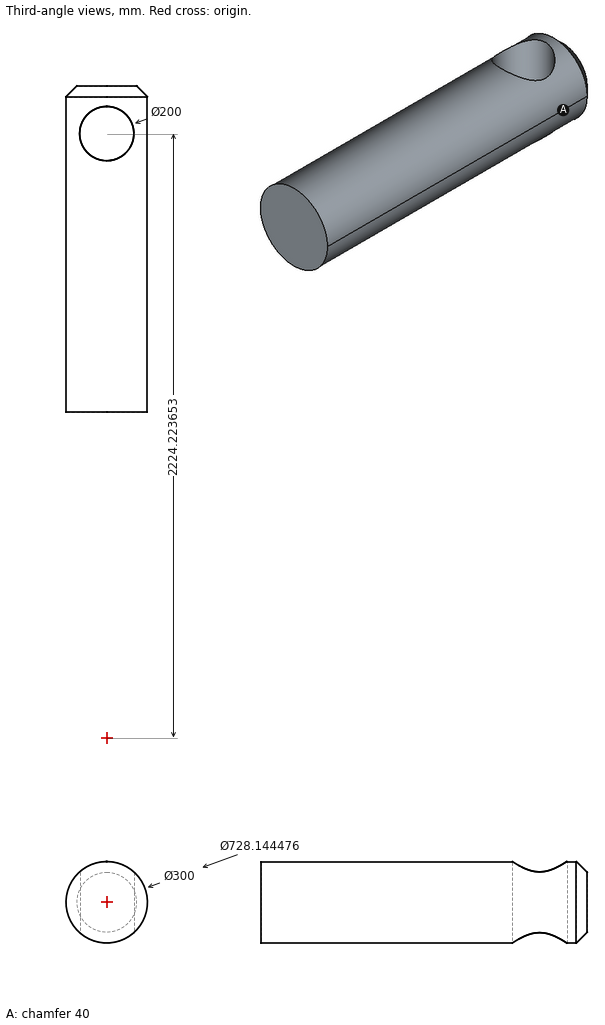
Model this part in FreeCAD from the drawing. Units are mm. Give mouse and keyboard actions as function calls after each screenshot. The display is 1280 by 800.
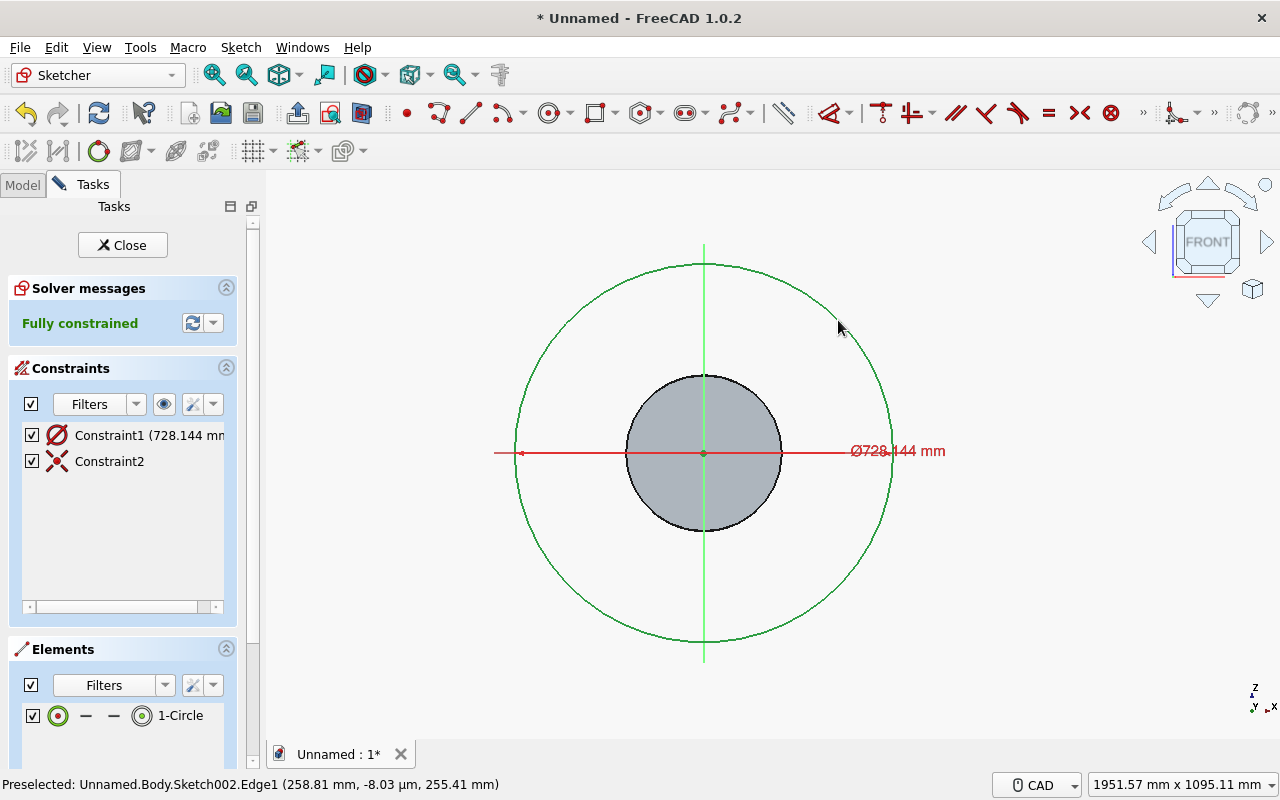
click(123, 245)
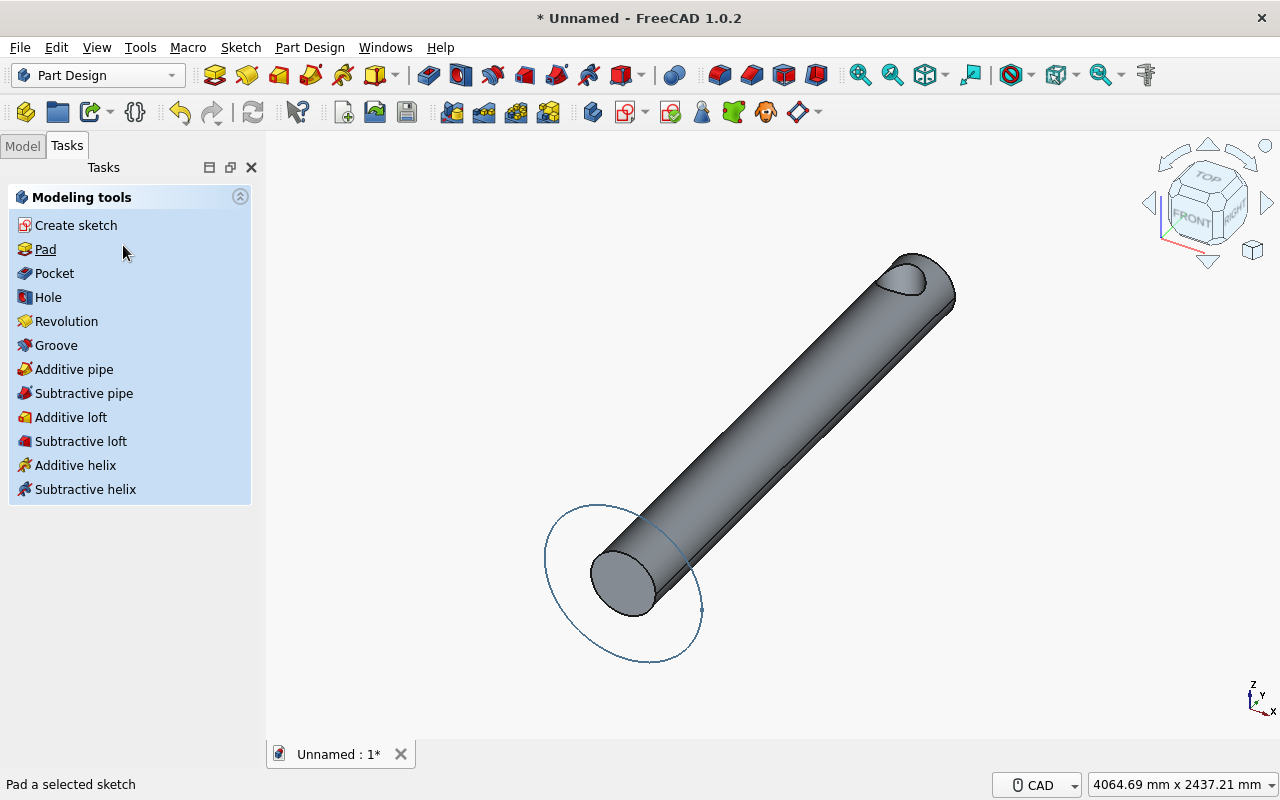
click(430, 76)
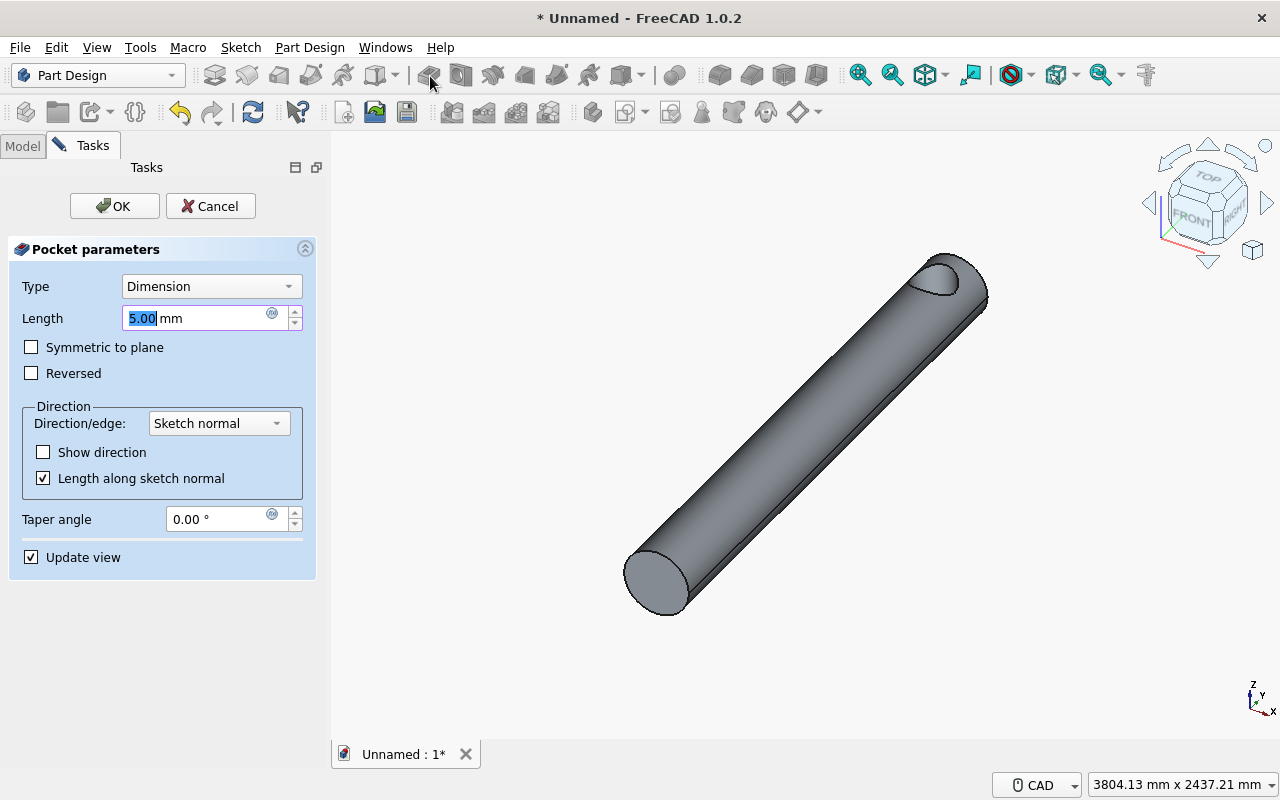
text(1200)
key(Tab)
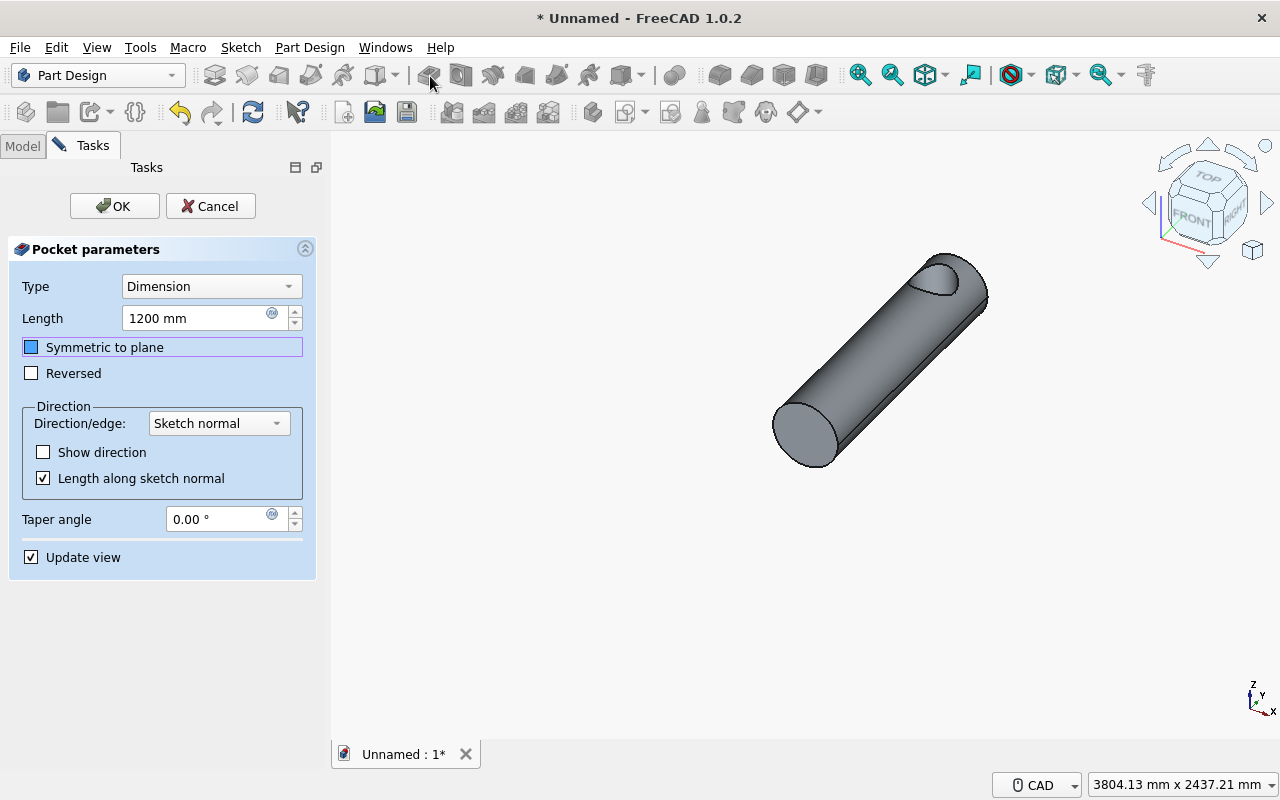
click(115, 206)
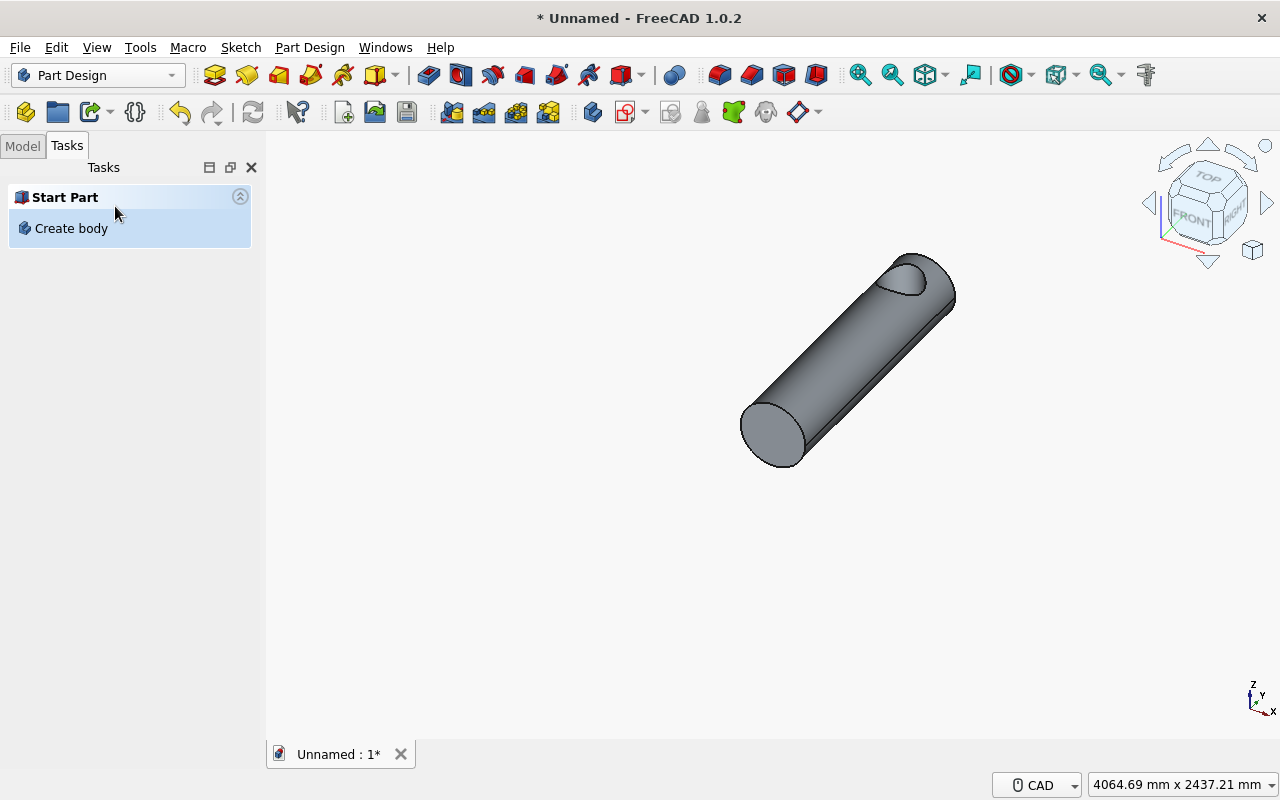
key(v)
key(f)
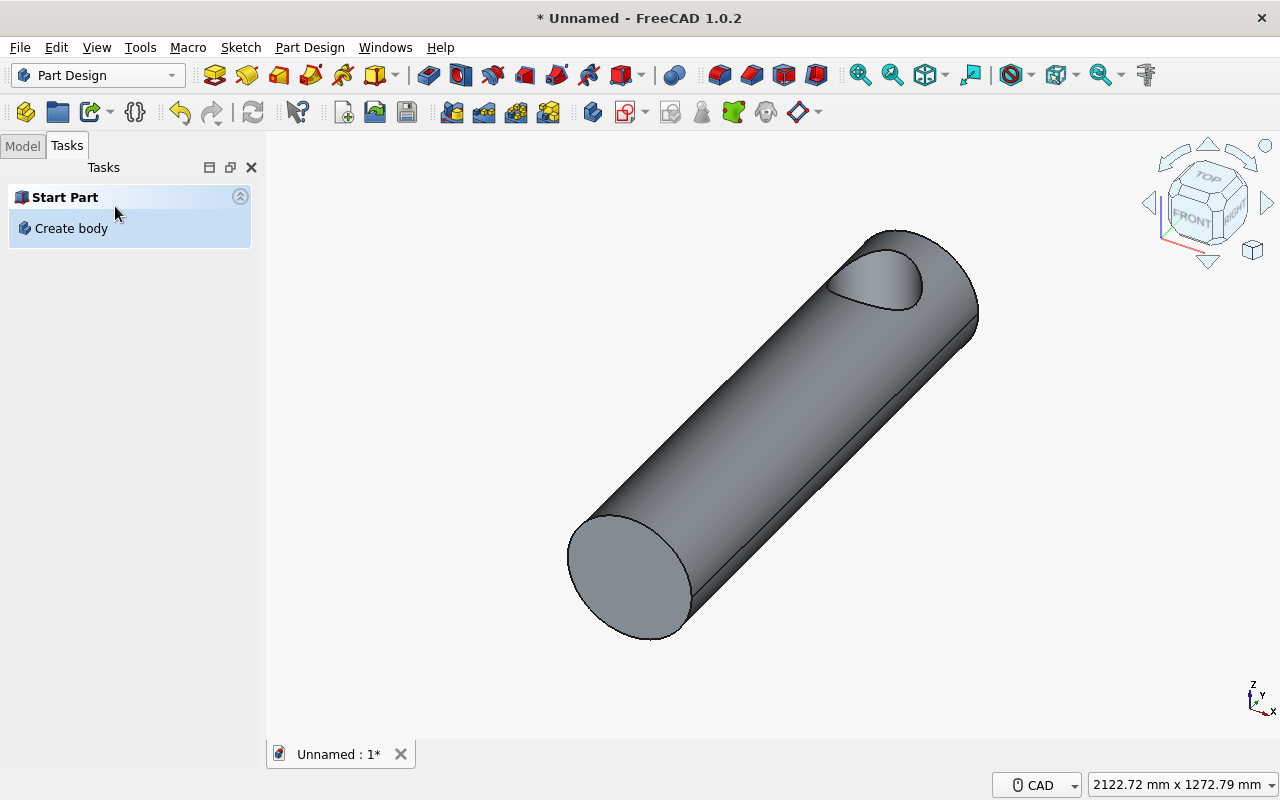
key(0)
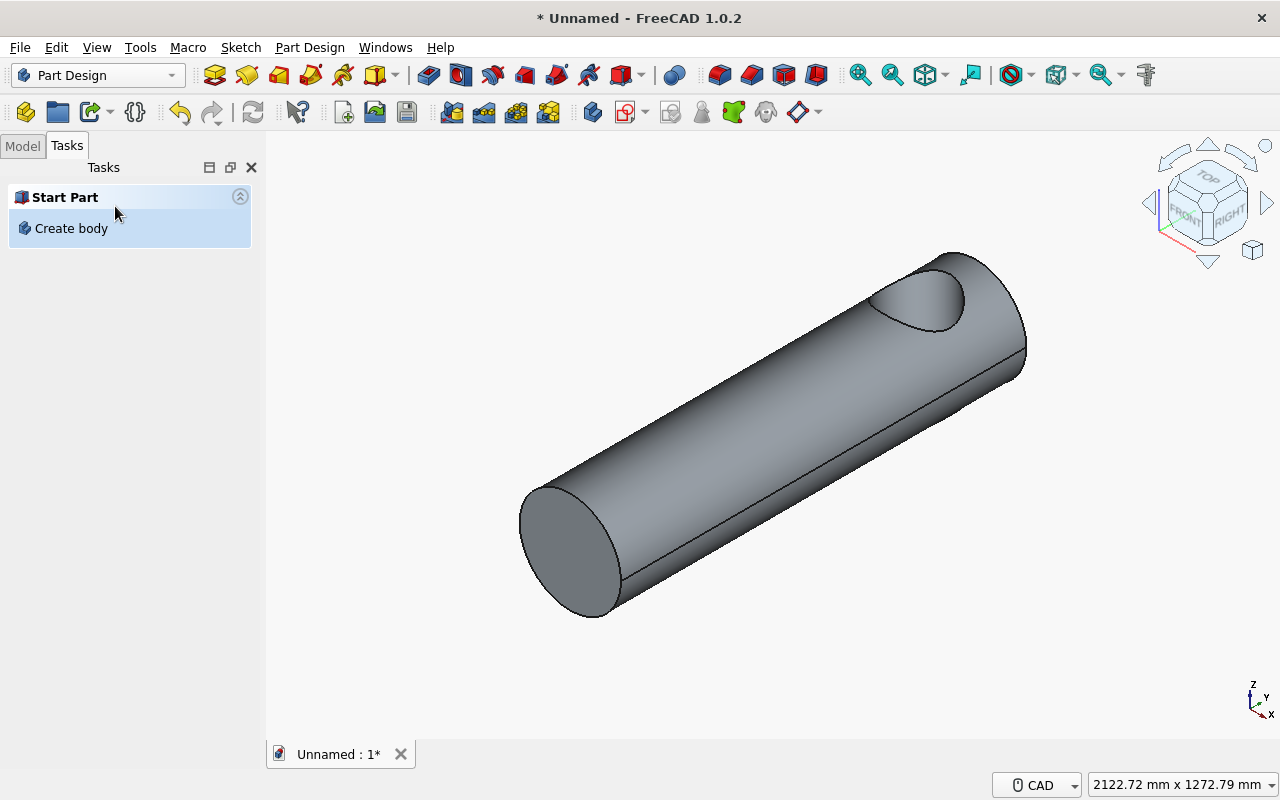
click(991, 270)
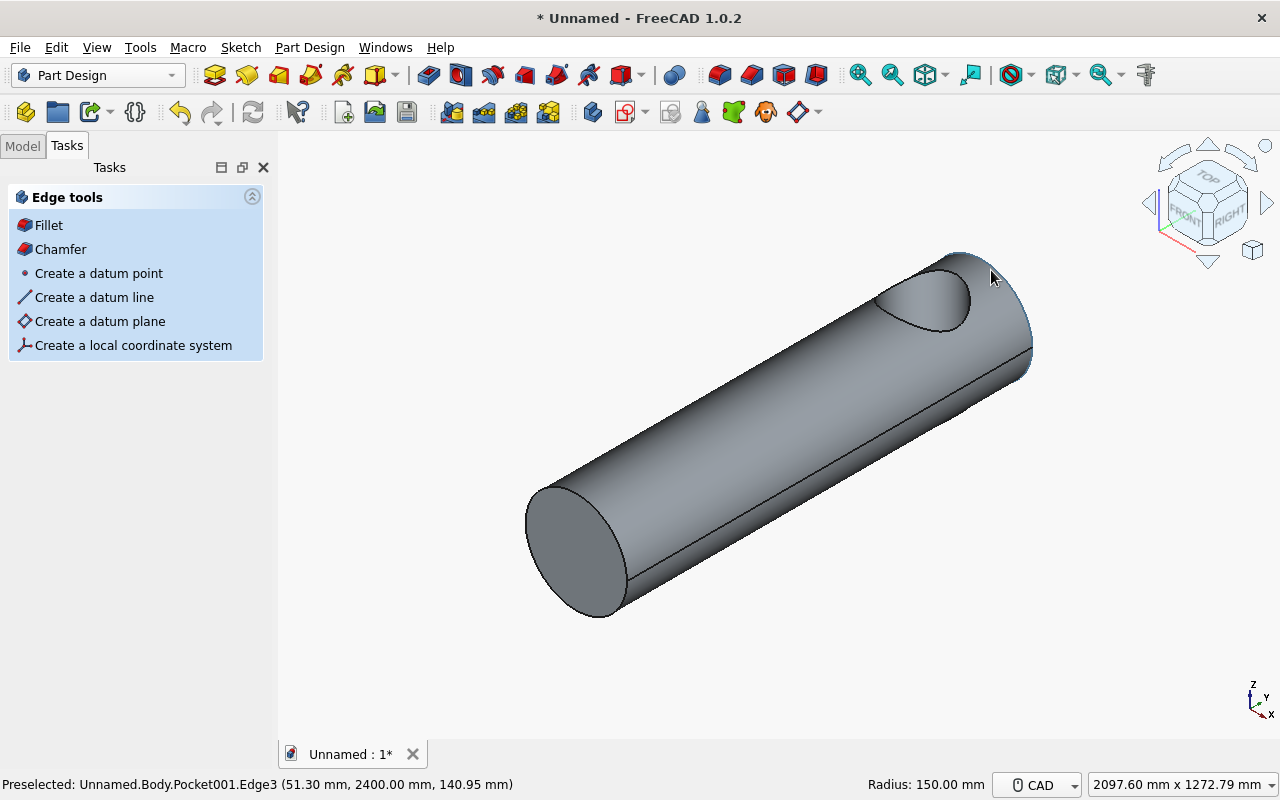
click(752, 76)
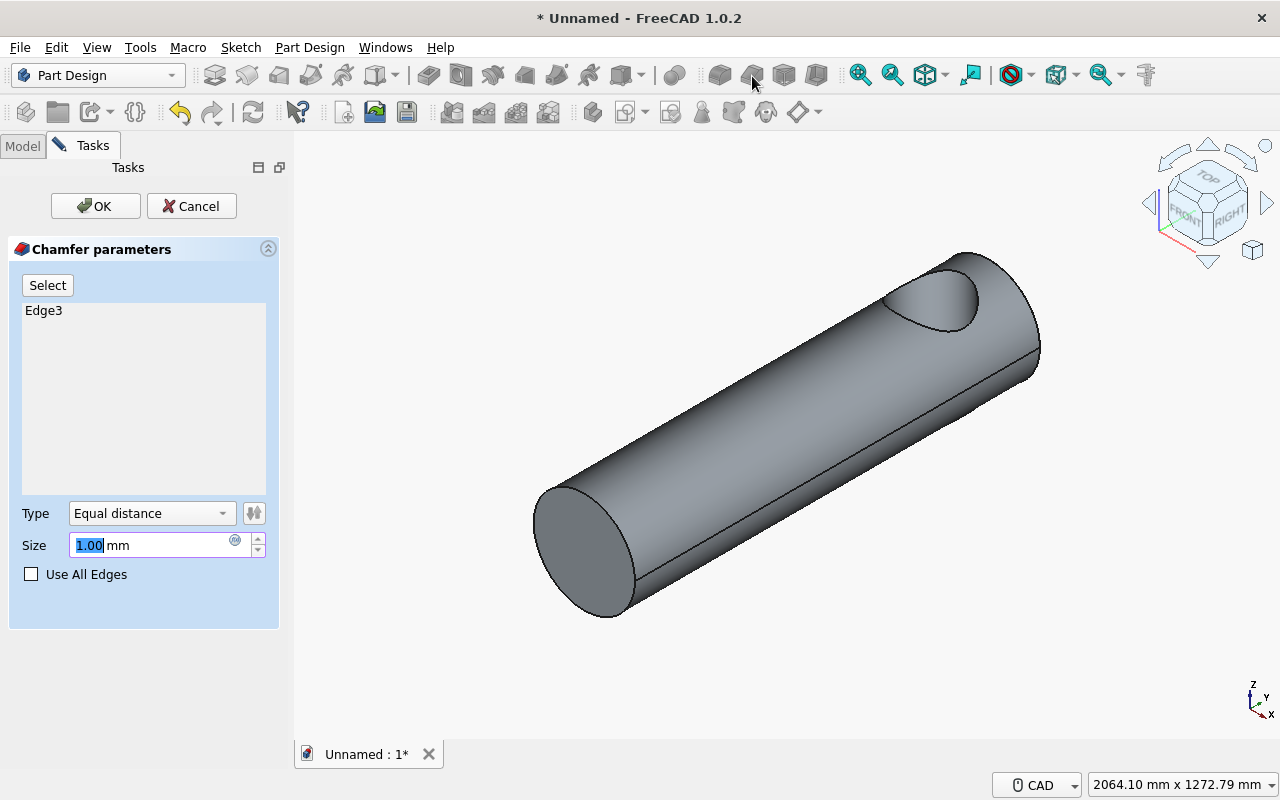
text(40)
key(Tab)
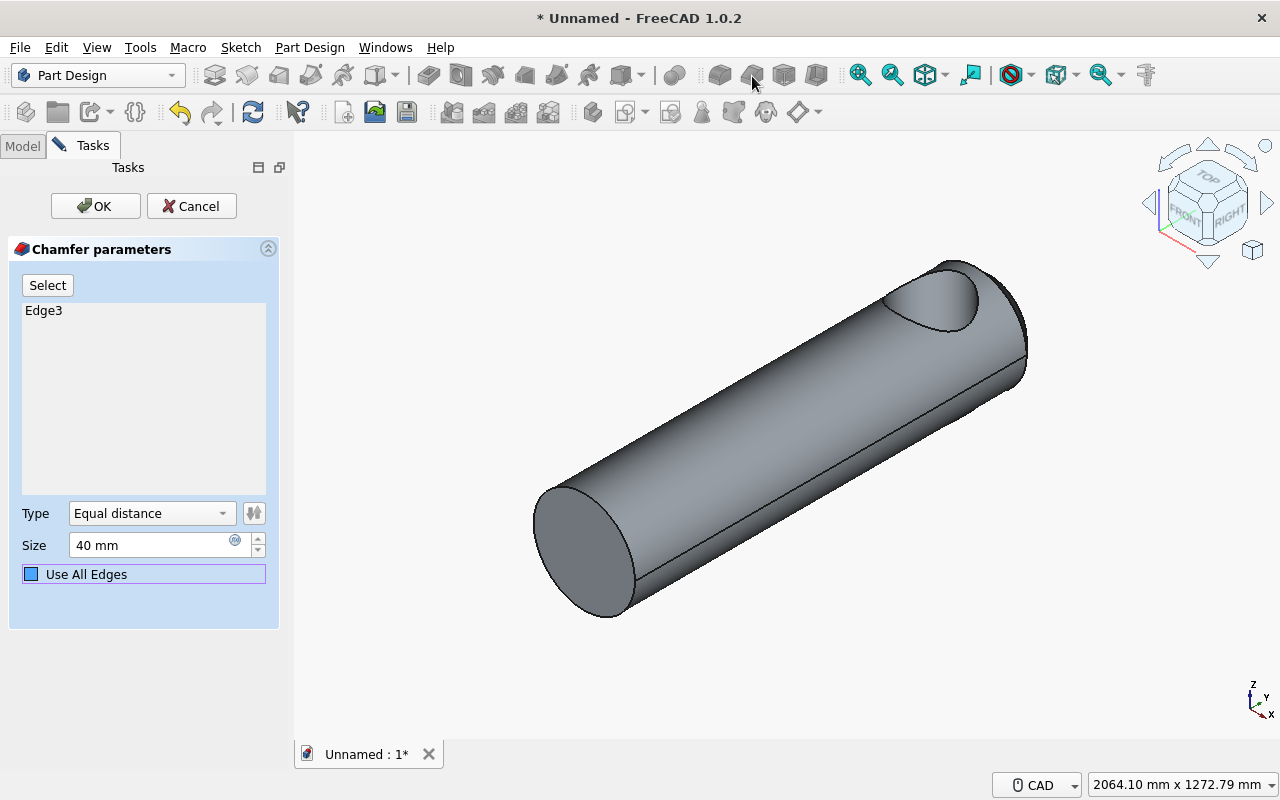
click(96, 206)